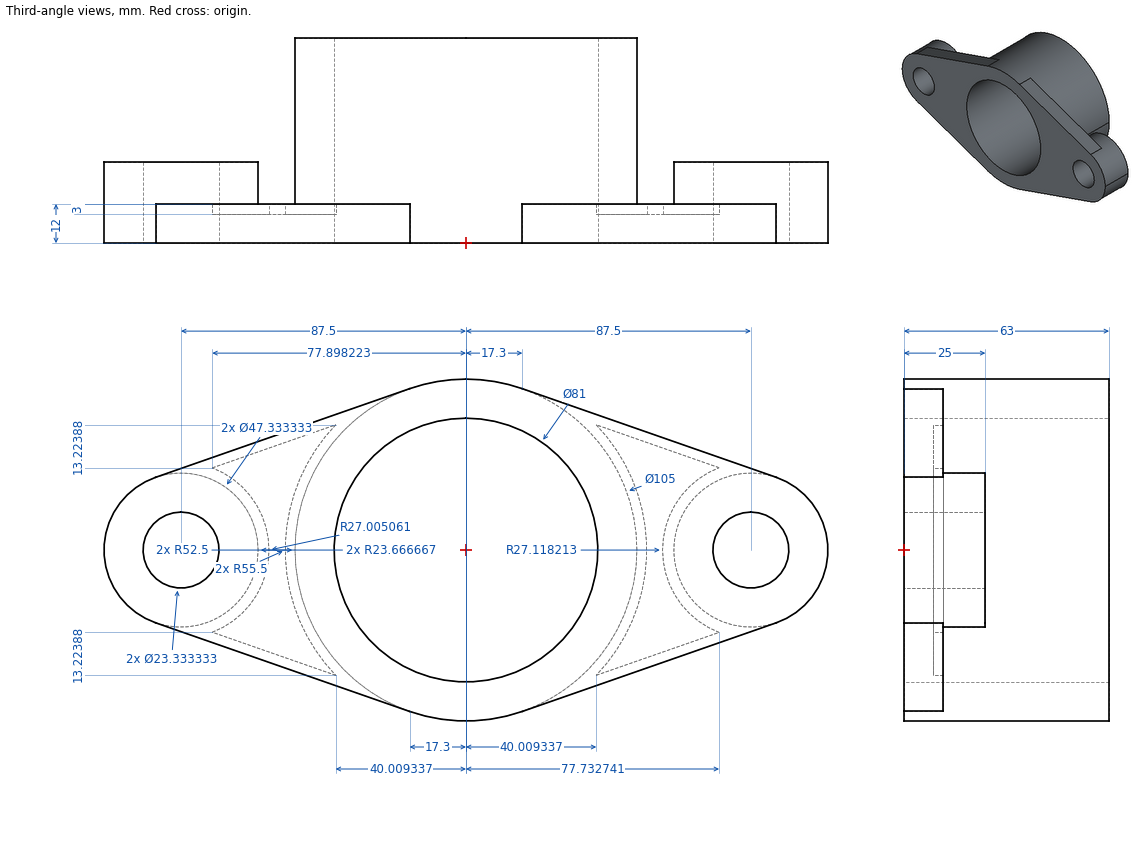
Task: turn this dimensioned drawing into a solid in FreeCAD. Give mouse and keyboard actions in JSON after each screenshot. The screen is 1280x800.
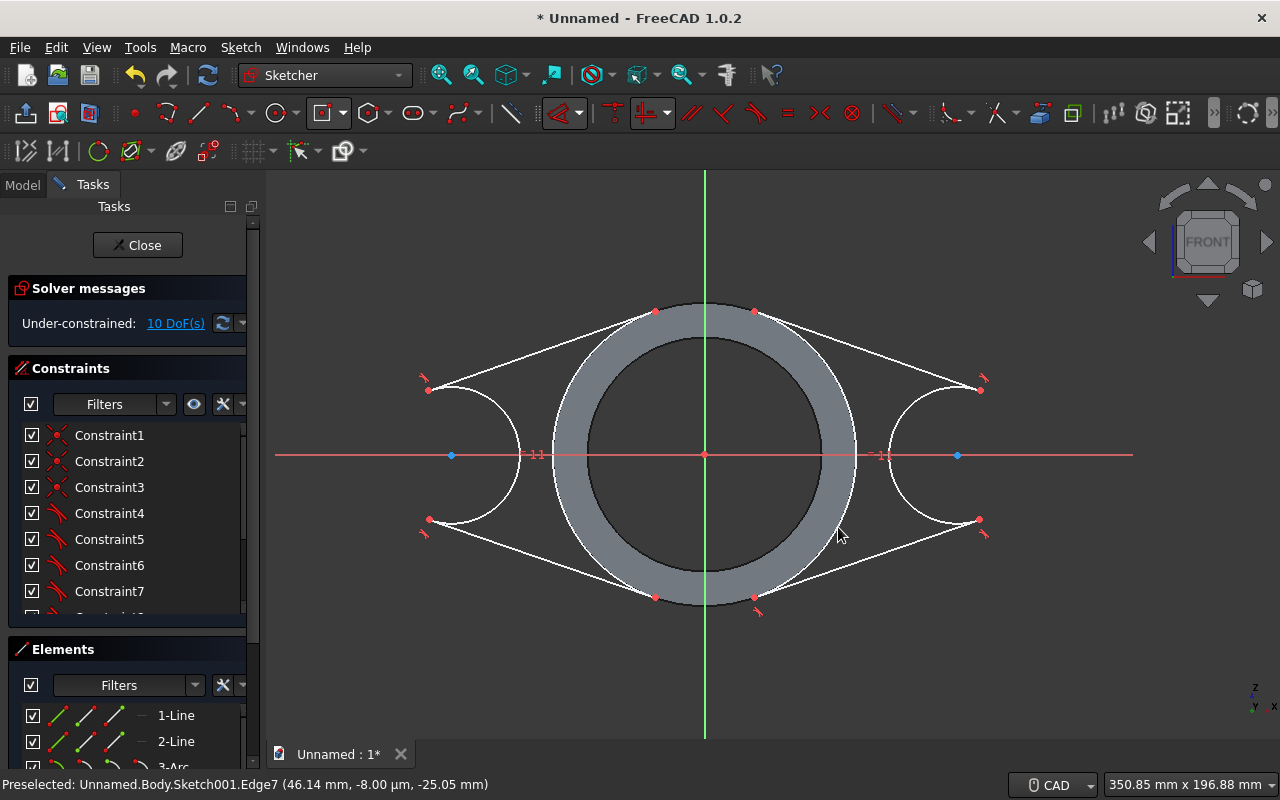
{"action": "left_click", "coordinate": [501, 502]}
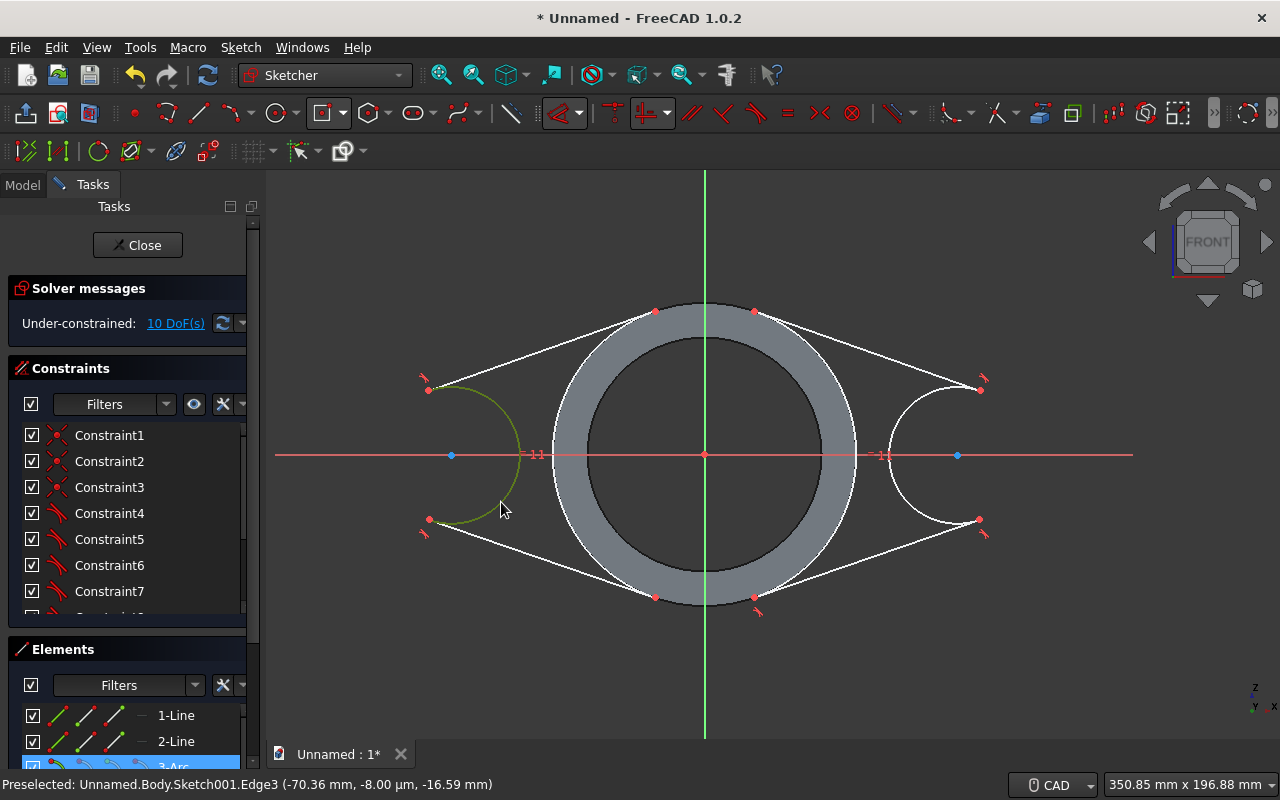
{"action": "left_click", "coordinate": [908, 408]}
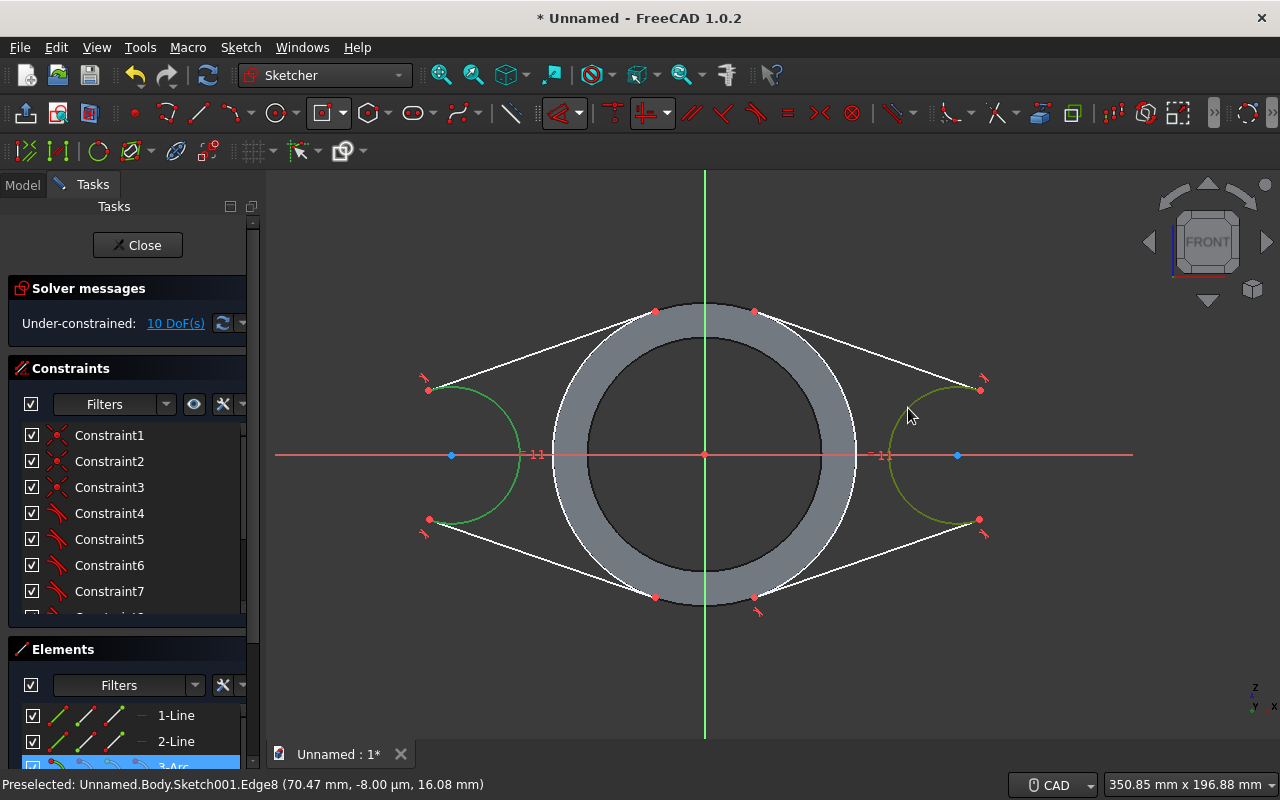
{"action": "key", "text": "e"}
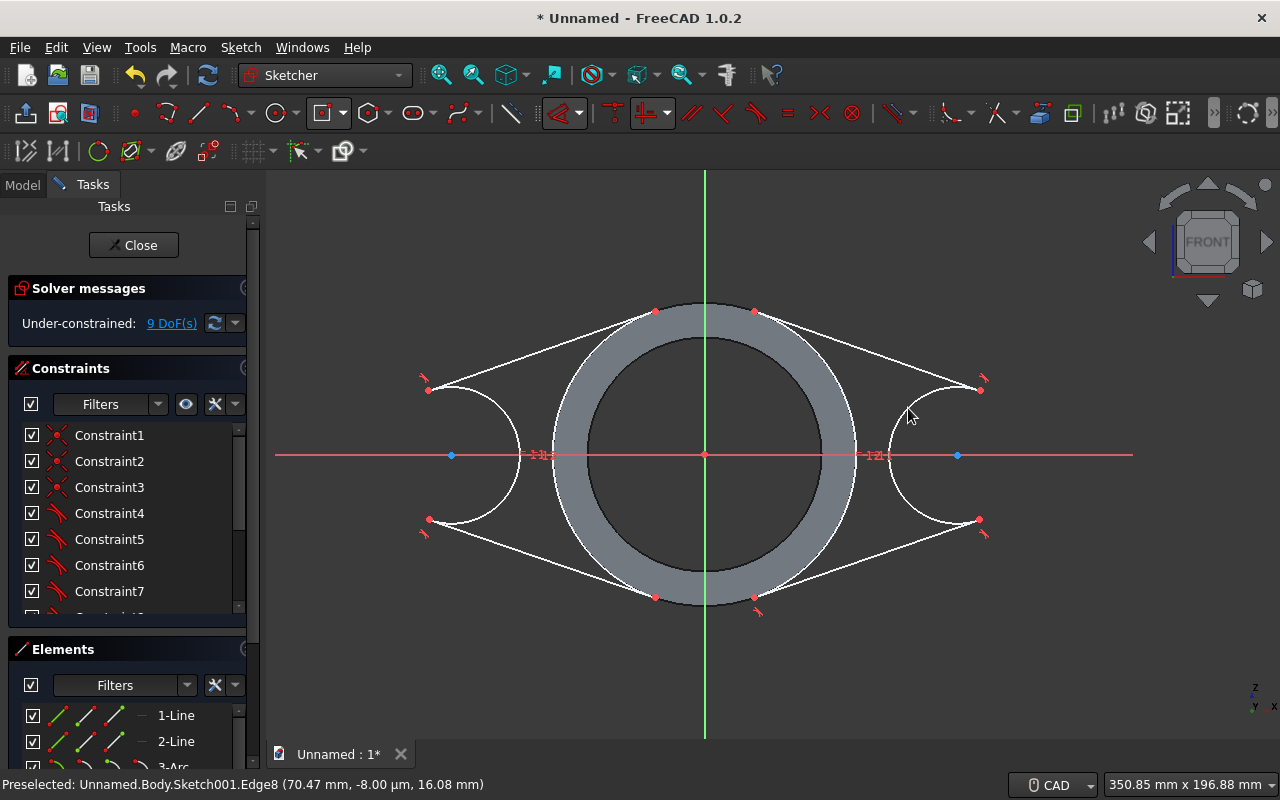
{"action": "left_click", "coordinate": [452, 455]}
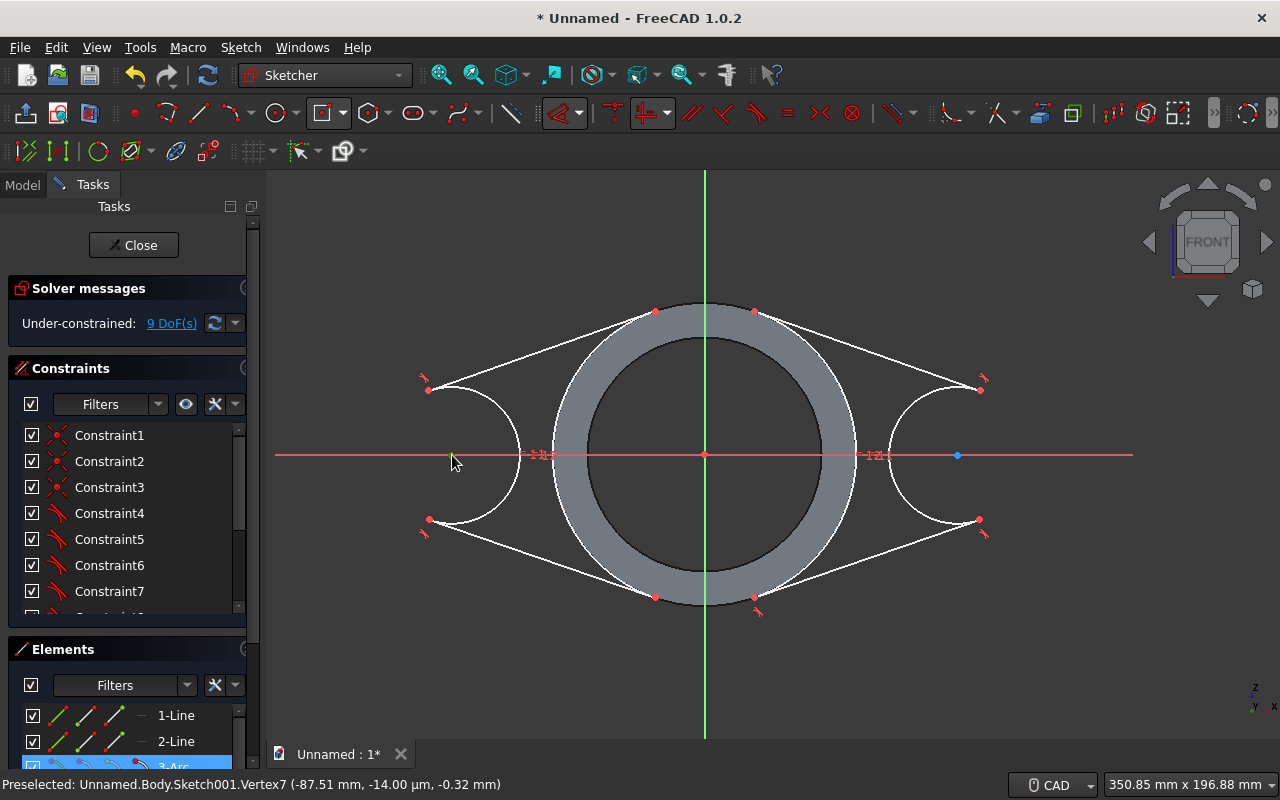
{"action": "left_click", "coordinate": [353, 455]}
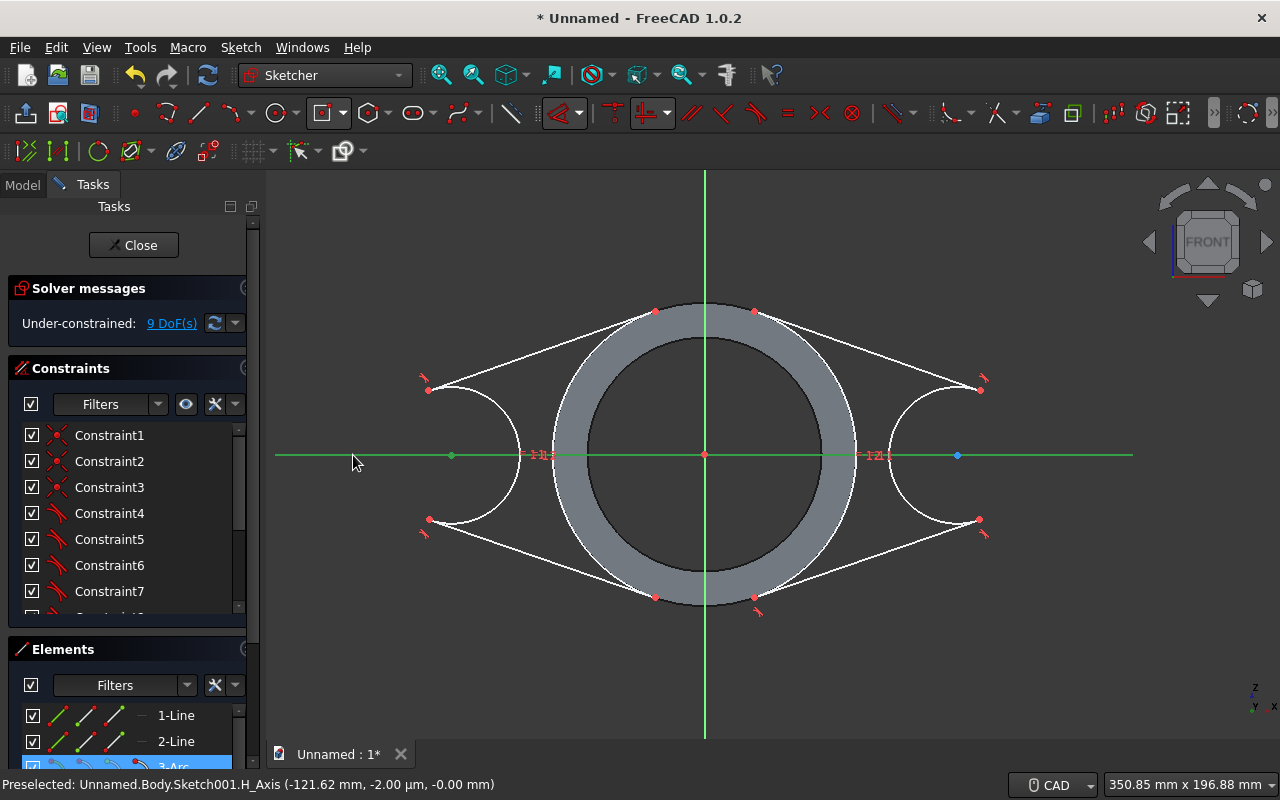
{"action": "key", "text": "c"}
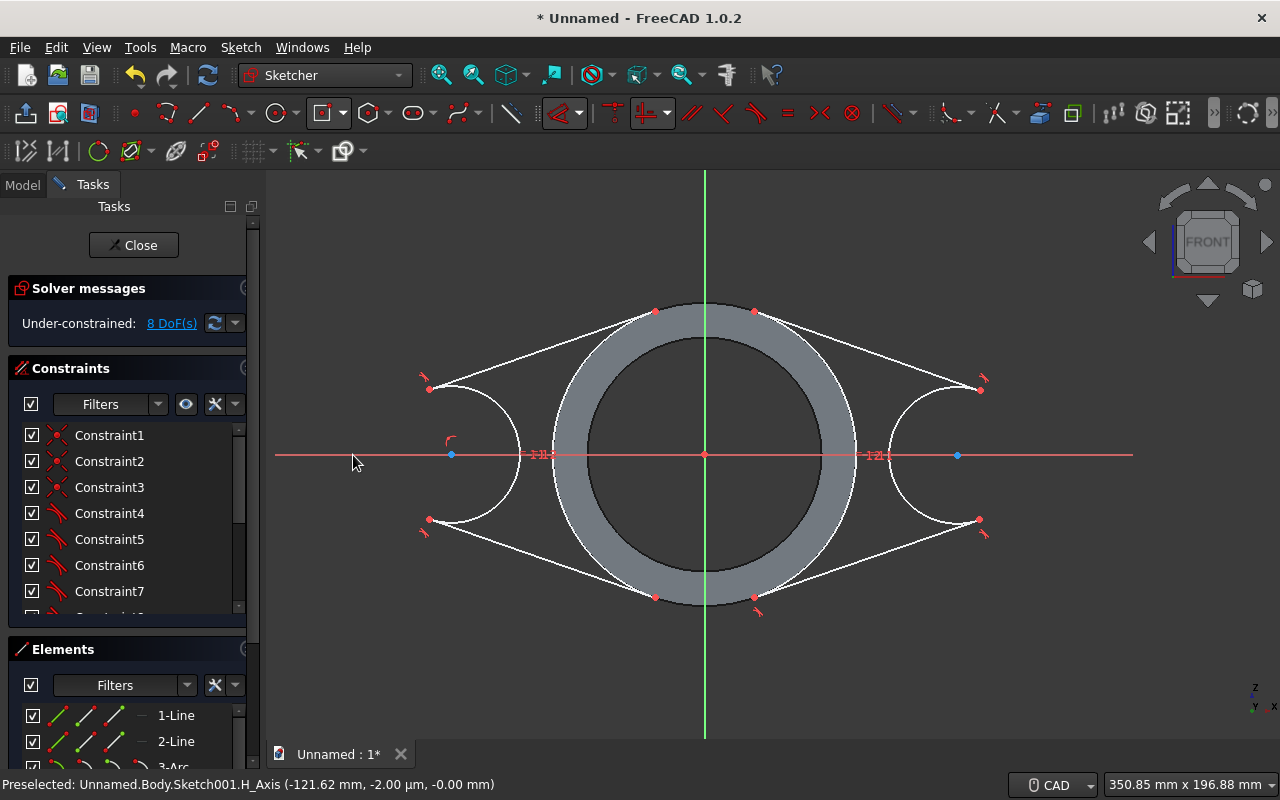
{"action": "left_click", "coordinate": [957, 455]}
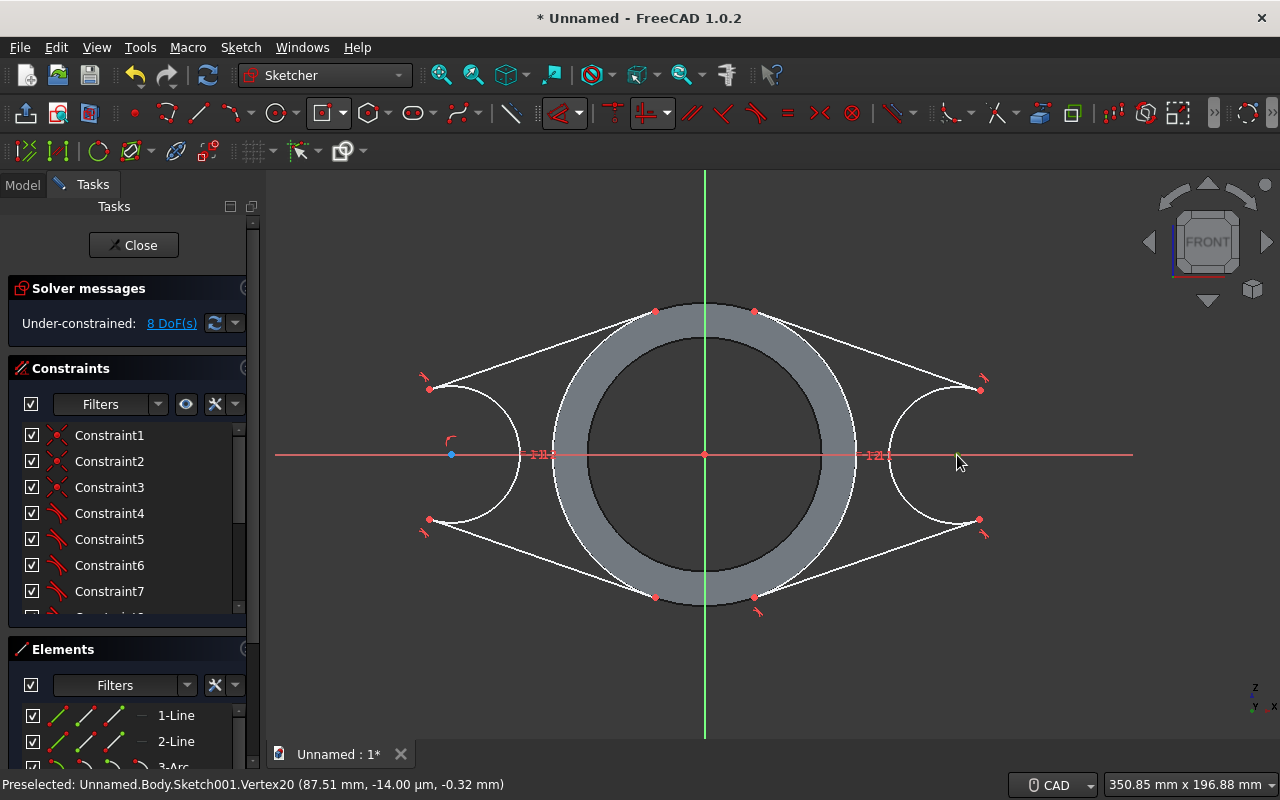
{"action": "left_click", "coordinate": [353, 455]}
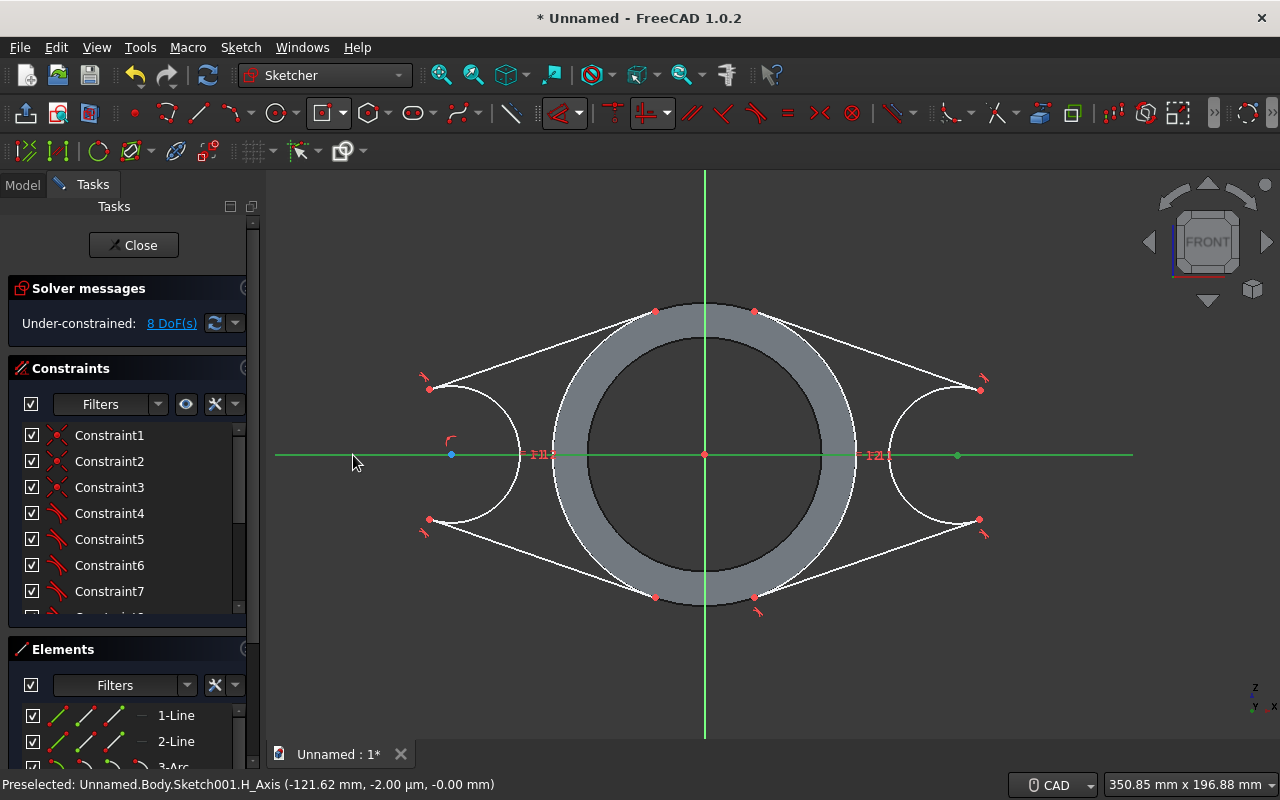
{"action": "key", "text": "c"}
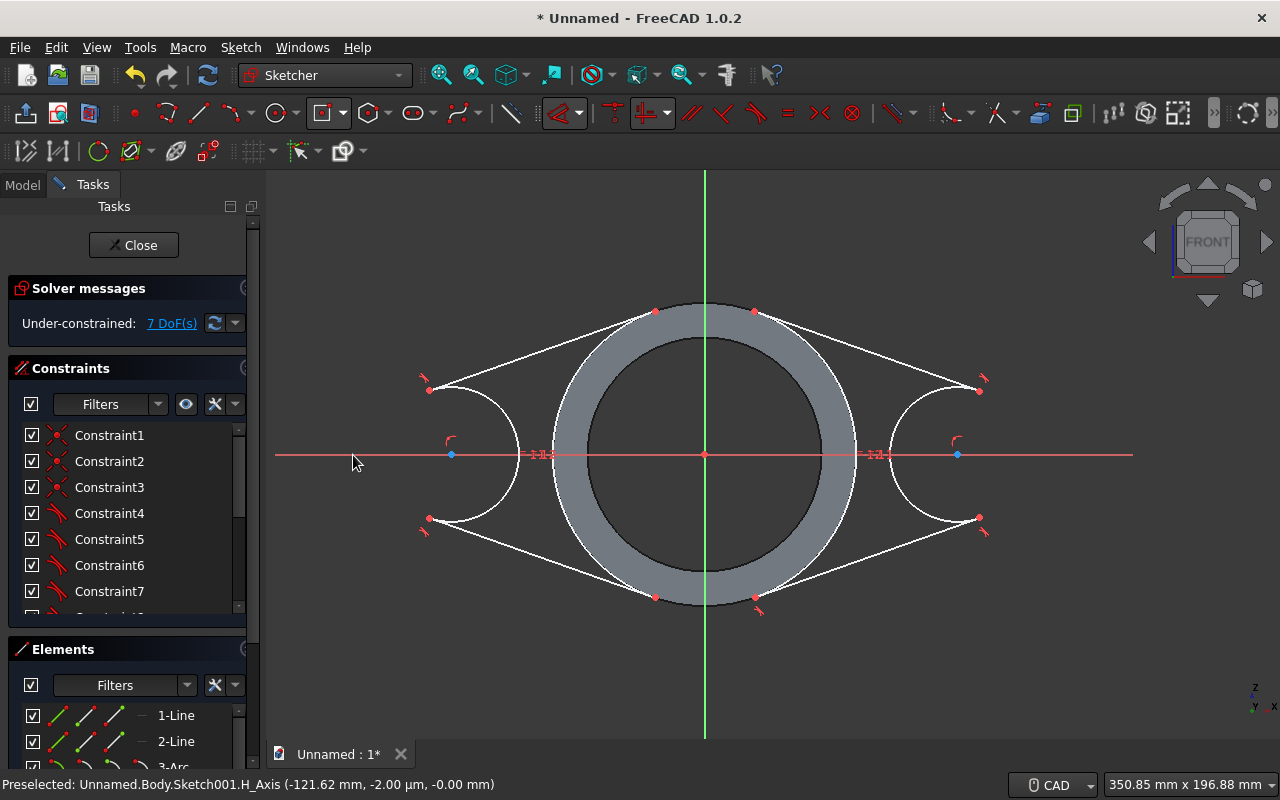
{"action": "left_click", "coordinate": [500, 501]}